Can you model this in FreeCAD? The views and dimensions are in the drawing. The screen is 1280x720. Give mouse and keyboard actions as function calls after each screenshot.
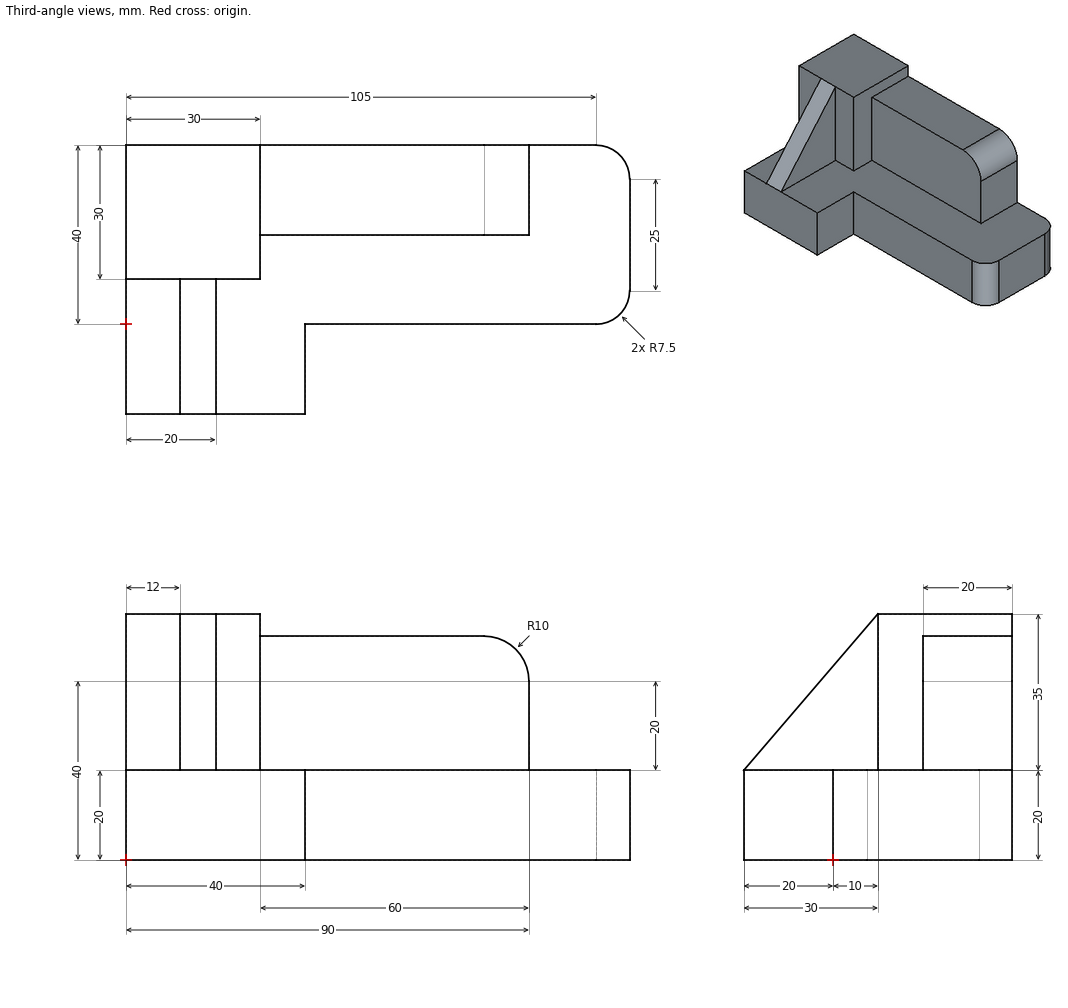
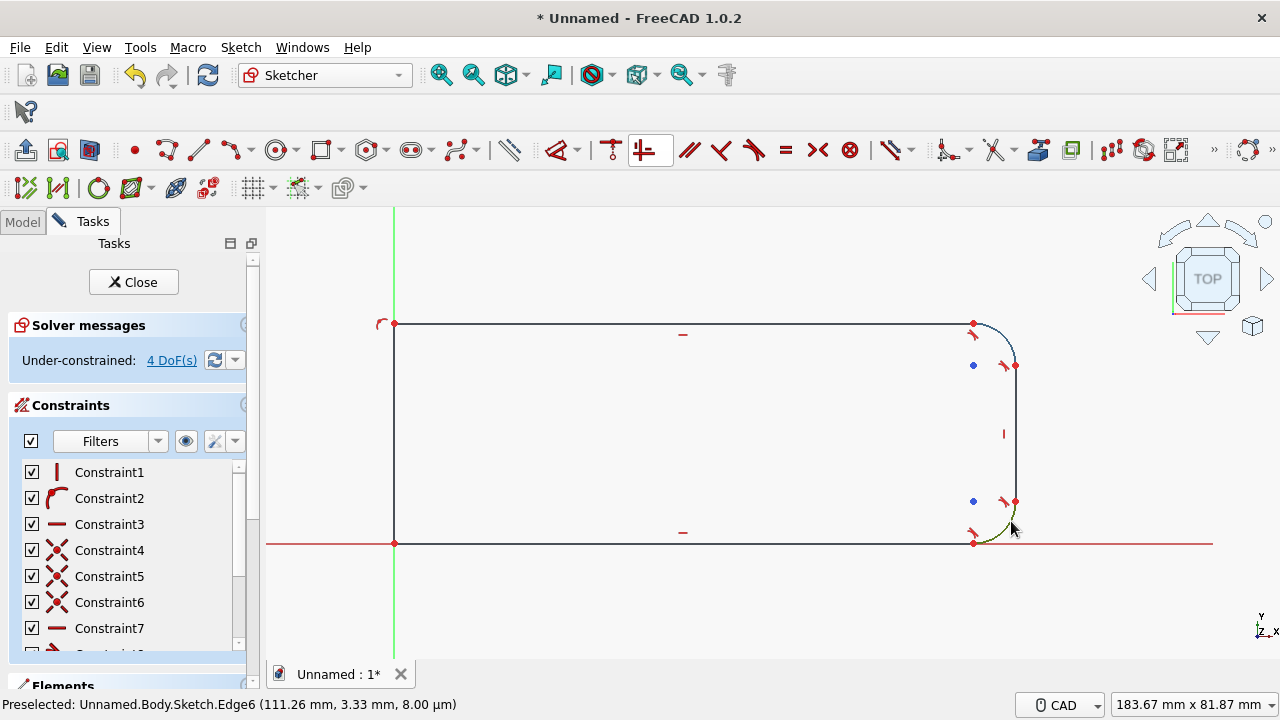
key(e)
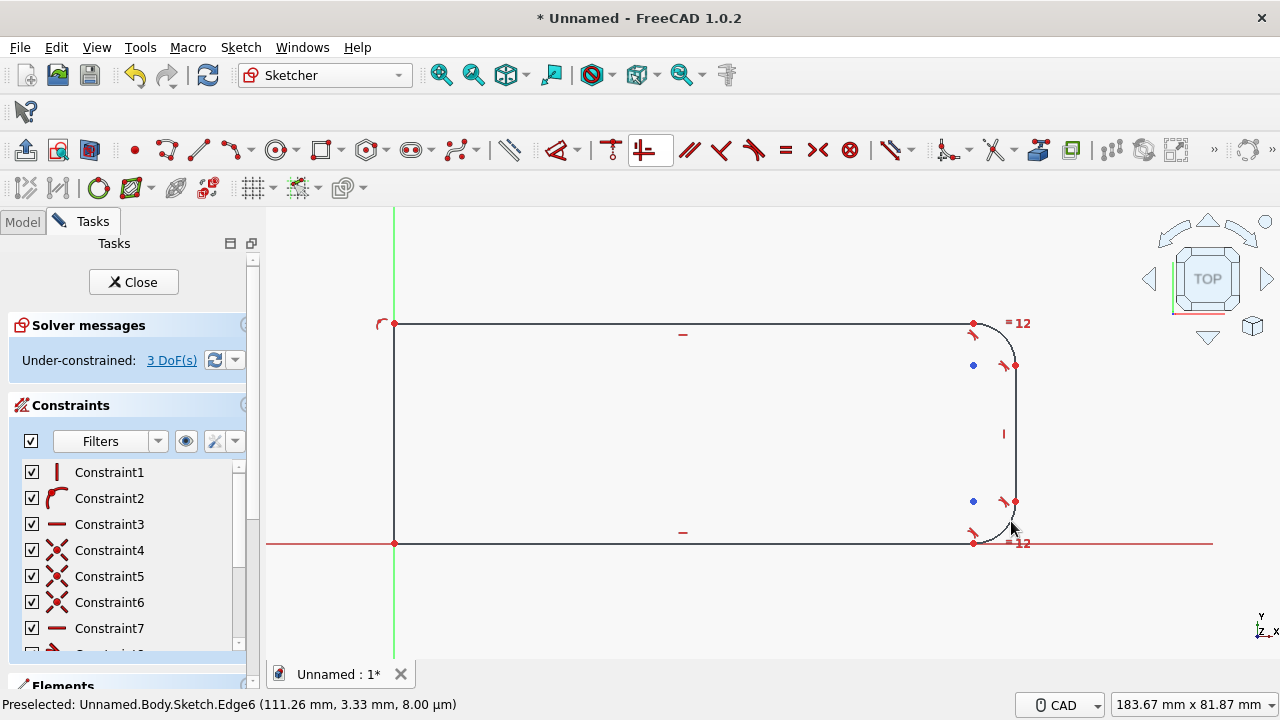
key(d)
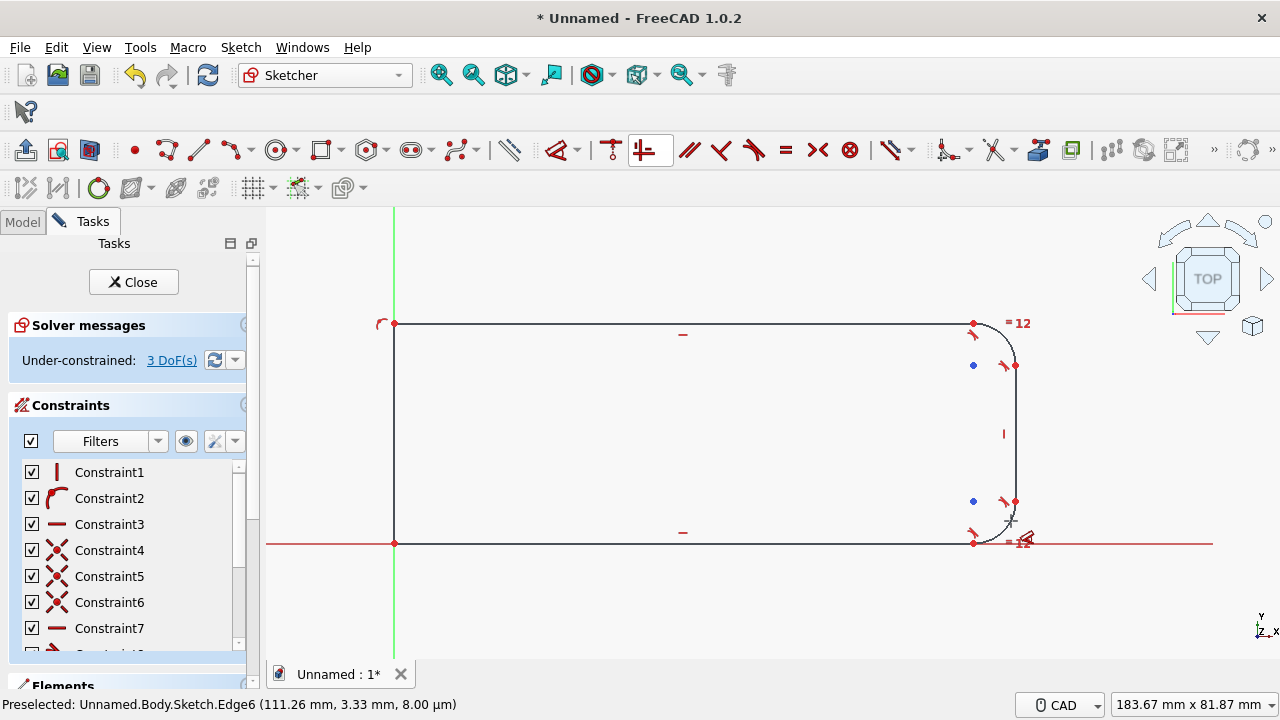
click(1011, 346)
click(1039, 331)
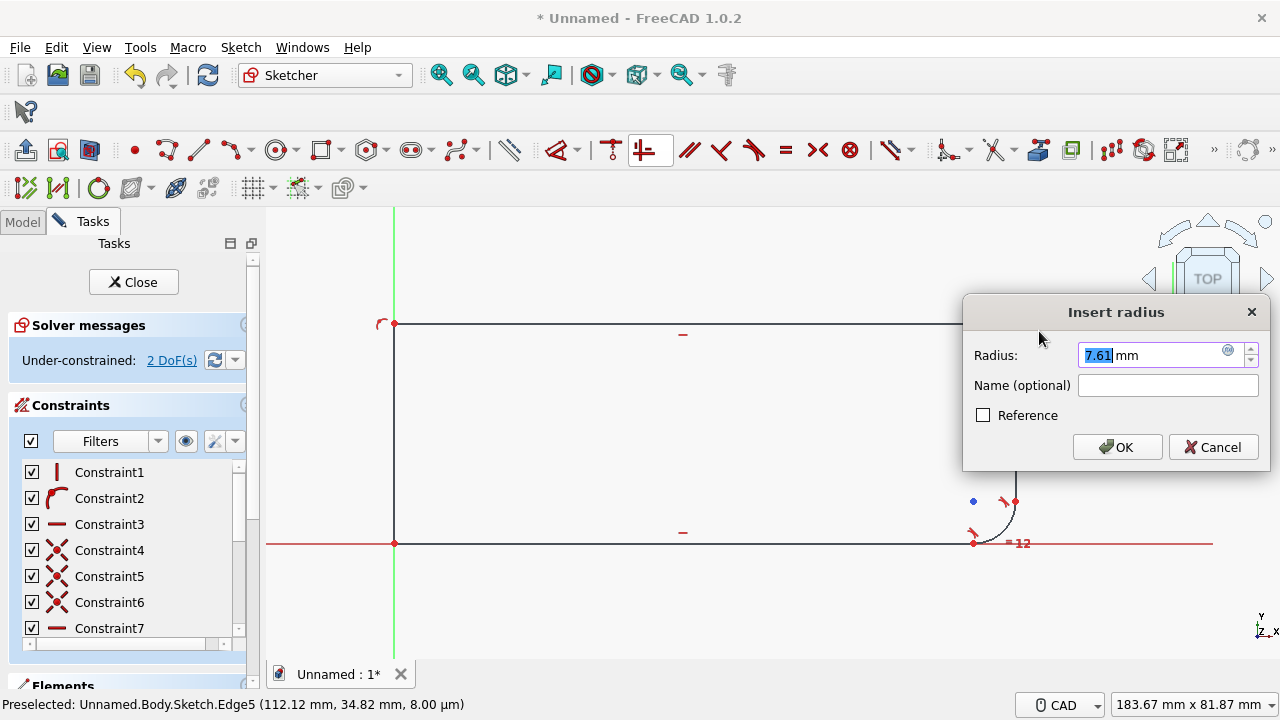
text(7.5)
key(Return)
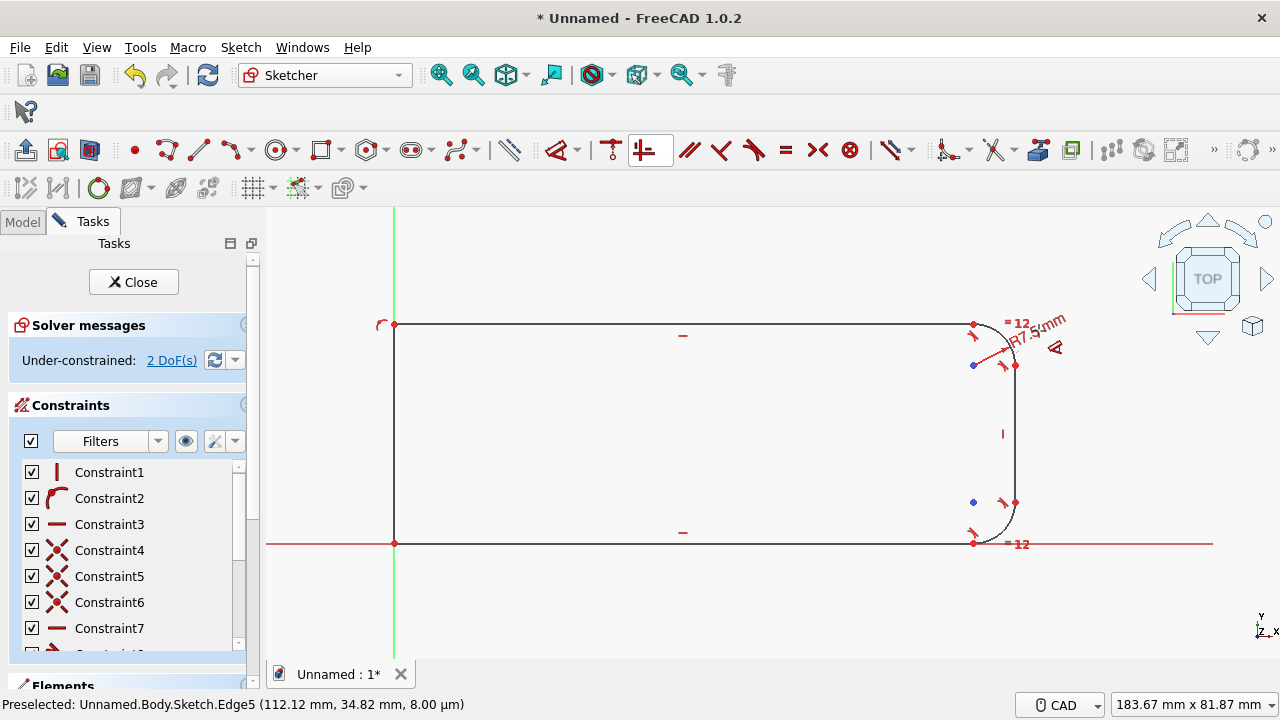
click(1015, 461)
click(1049, 434)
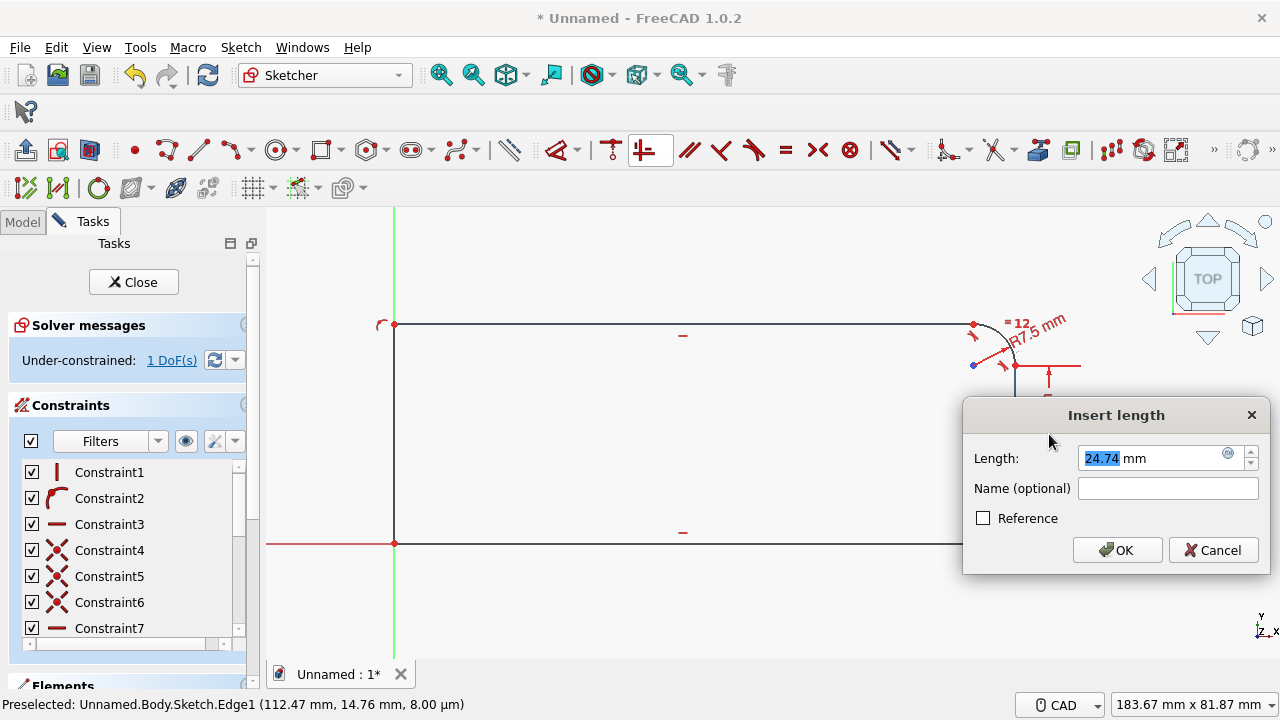
text(25)
key(Return)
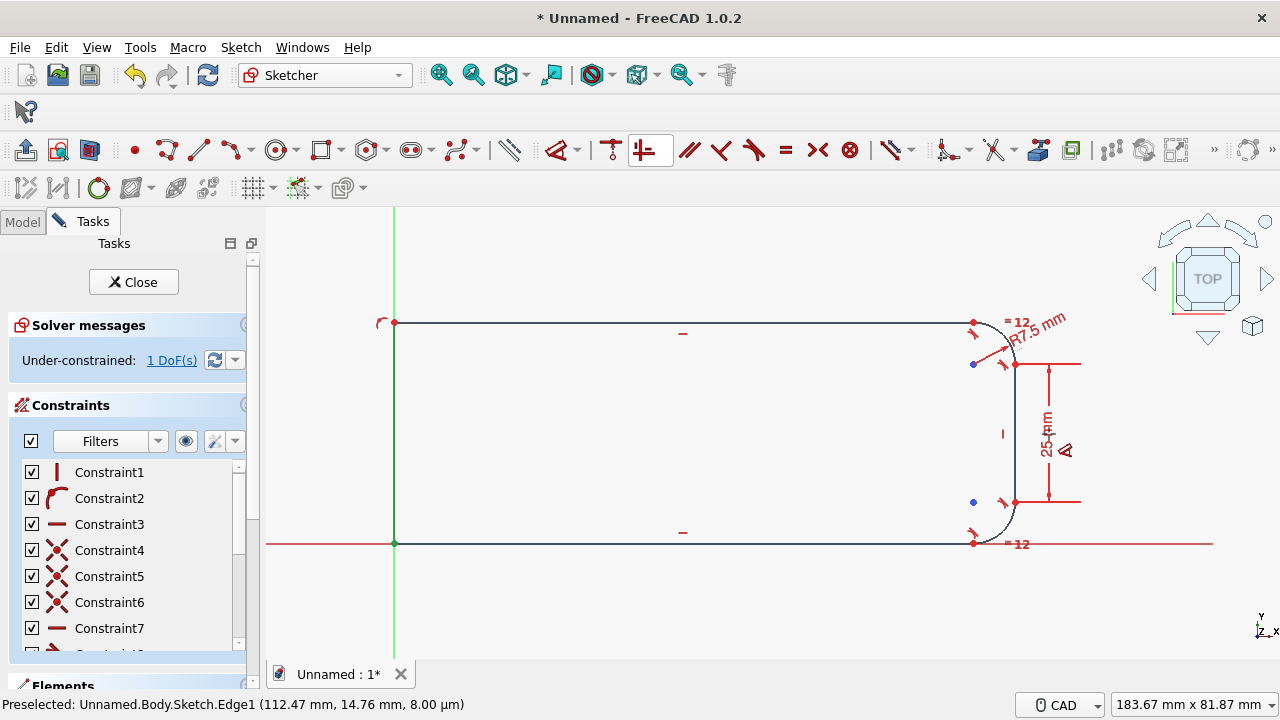
click(800, 323)
click(684, 289)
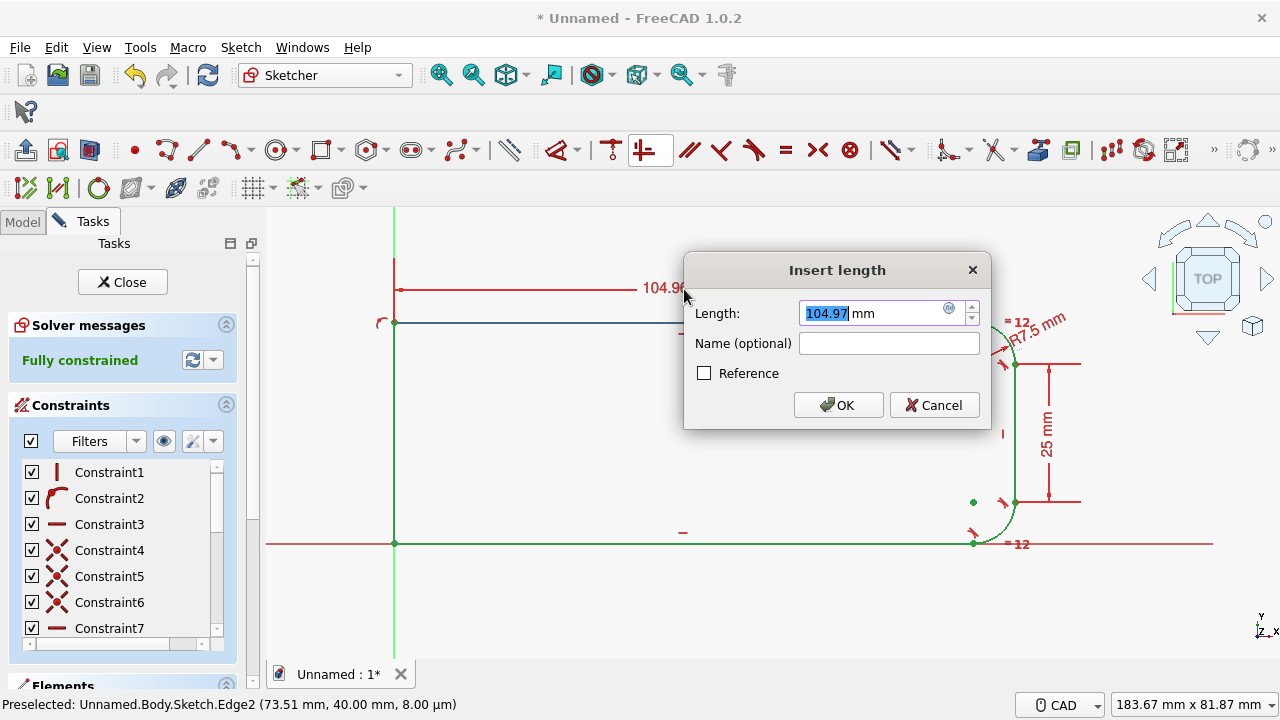
text(105)
key(Return)
key(Escape)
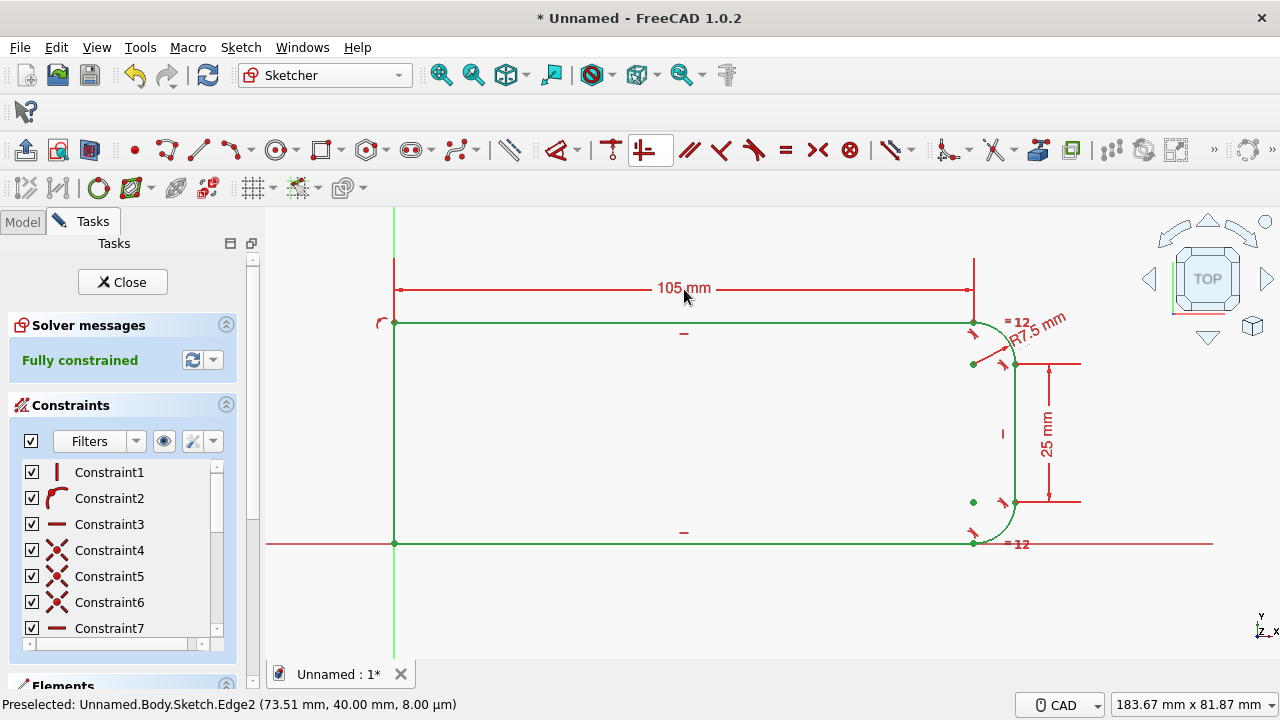
click(123, 282)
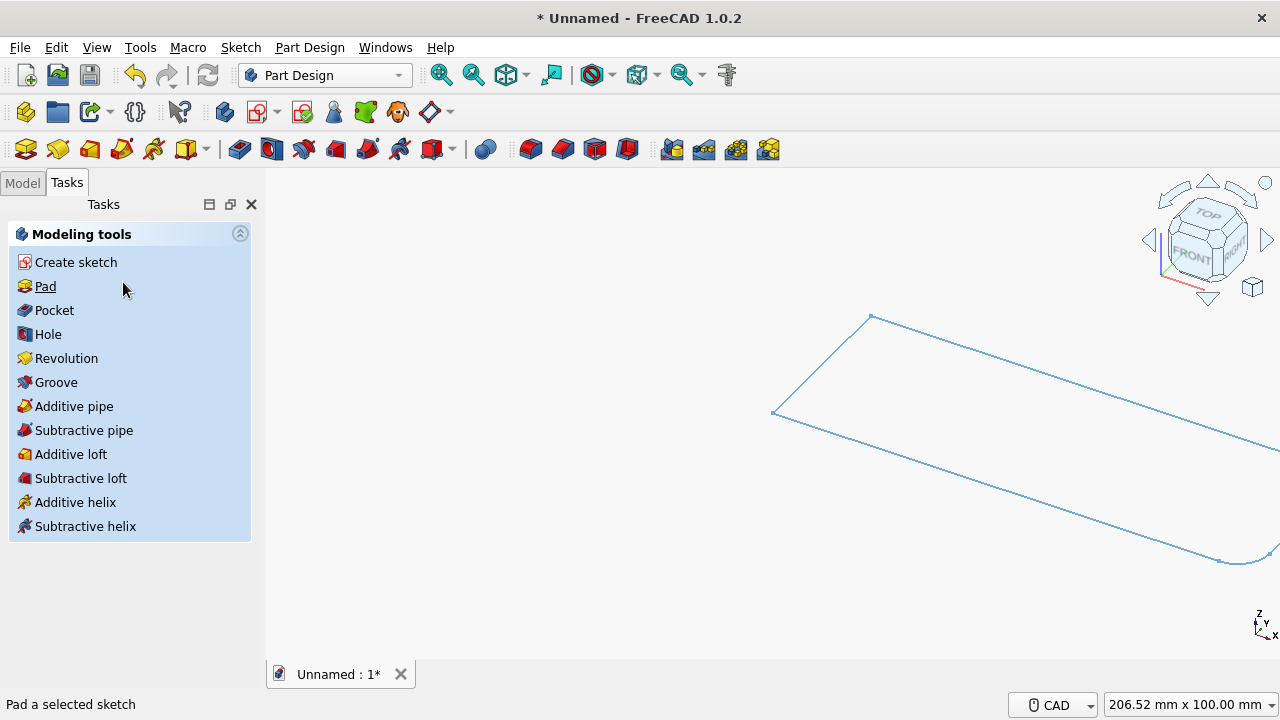
click(26, 150)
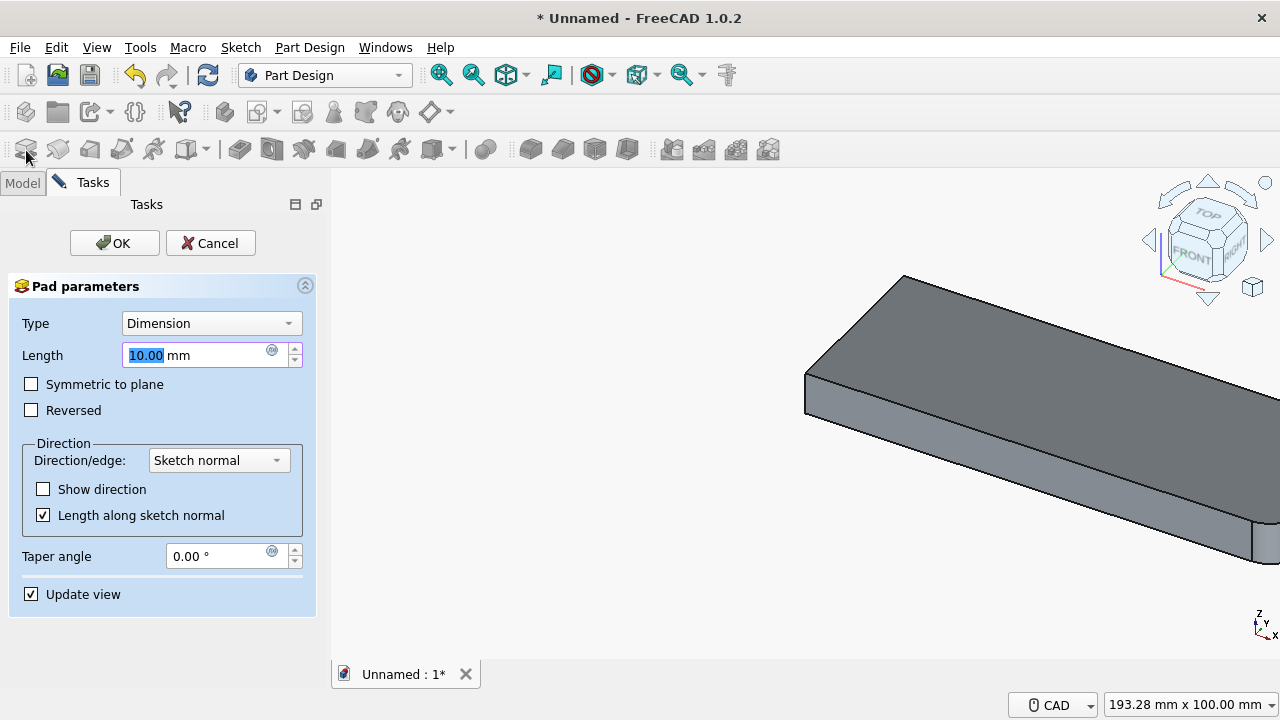
text(20)
key(Tab)